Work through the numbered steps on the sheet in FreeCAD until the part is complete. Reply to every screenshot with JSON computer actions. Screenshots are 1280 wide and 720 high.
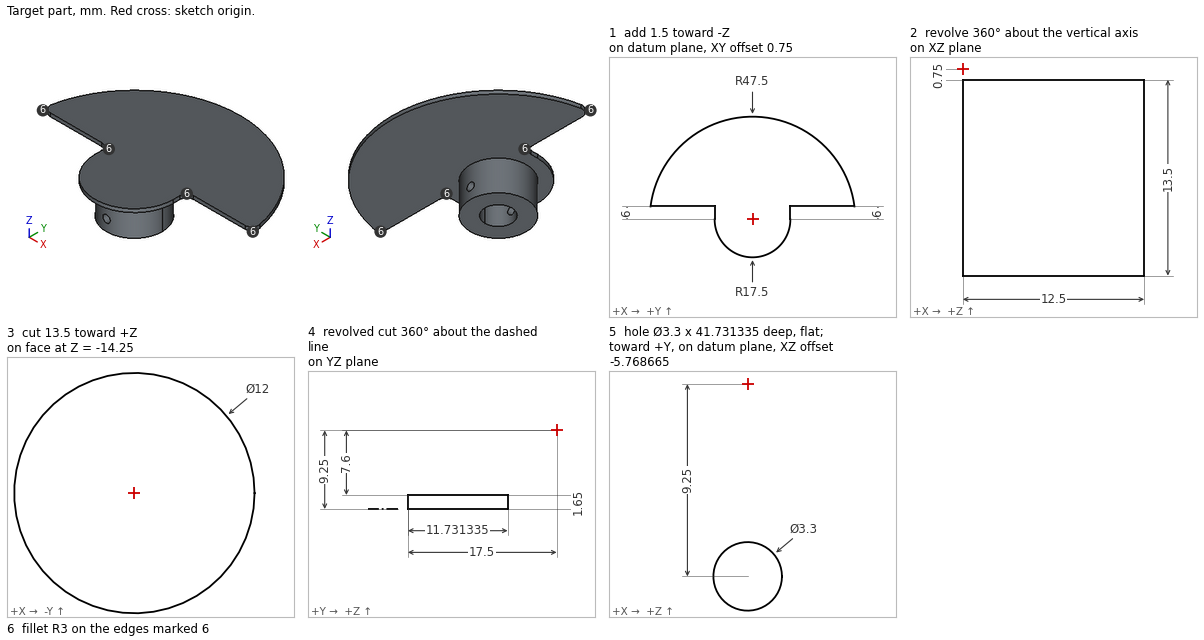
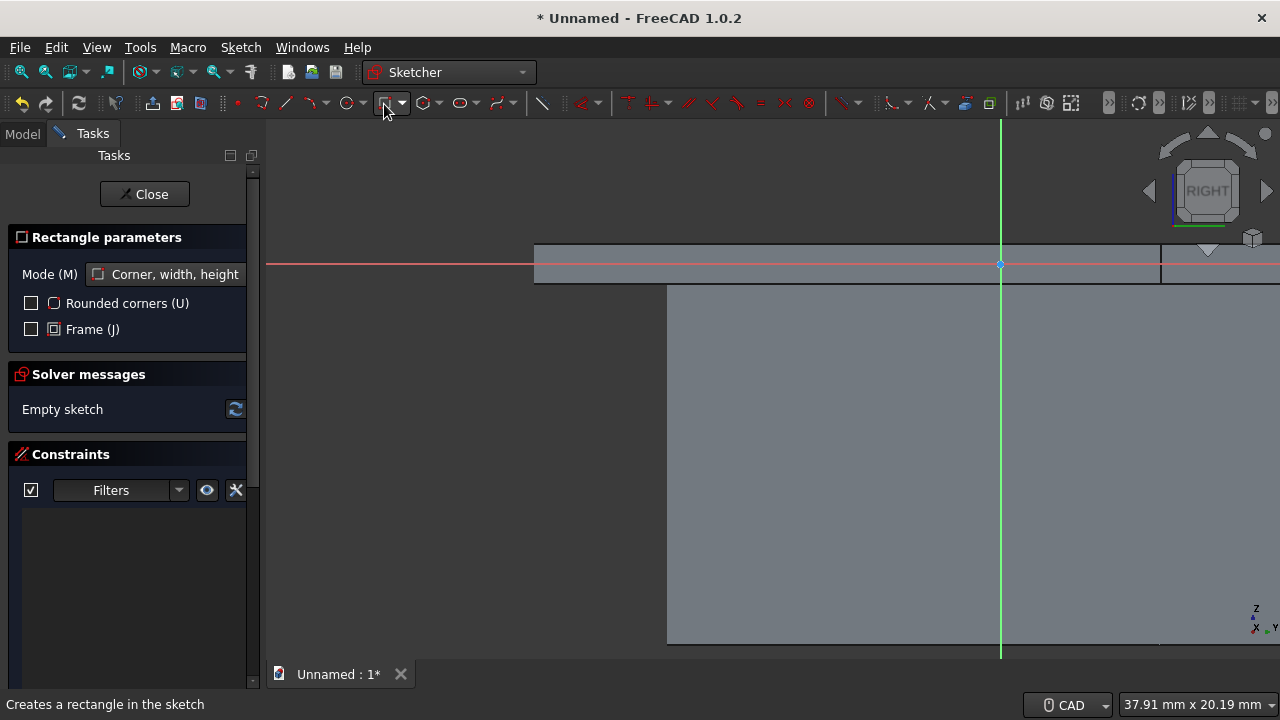
{"action": "left_click", "coordinate": [532, 468]}
{"action": "mouse_move", "coordinate": [846, 512]}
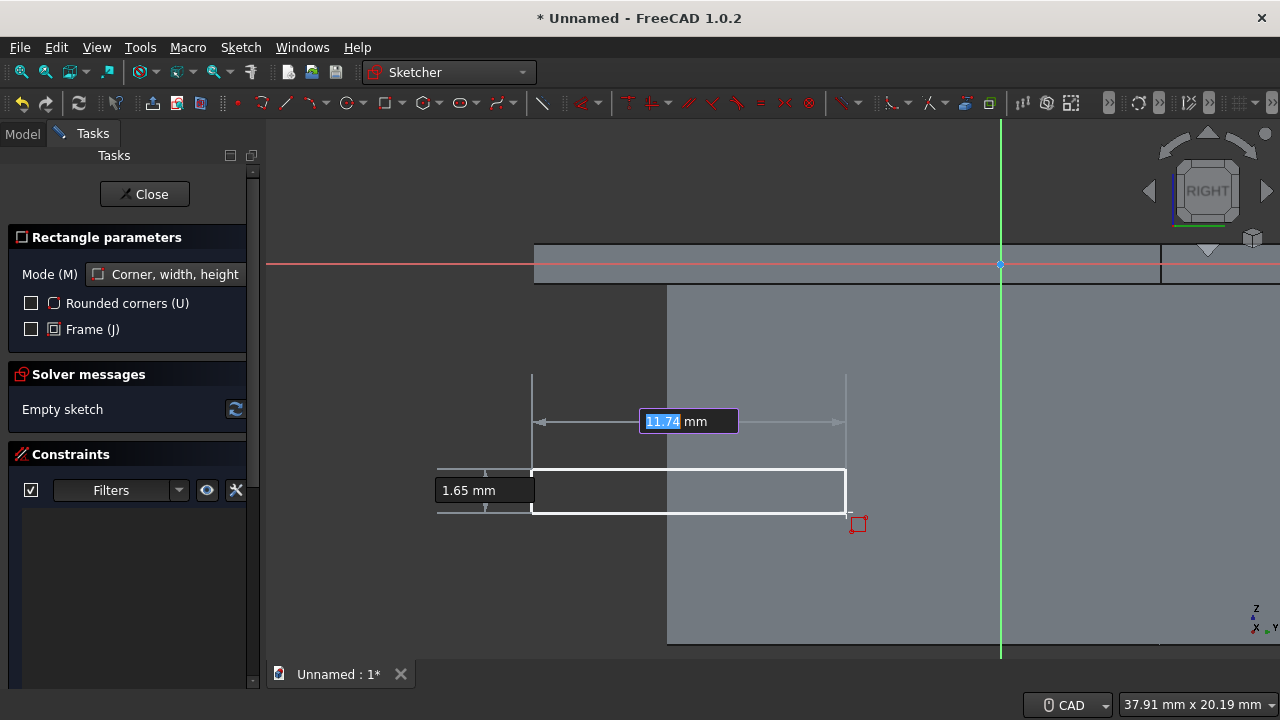
{"action": "type", "text": "11.731335"}
{"action": "key", "text": "Tab"}
{"action": "type", "text": "1.65"}
{"action": "key", "text": "Return"}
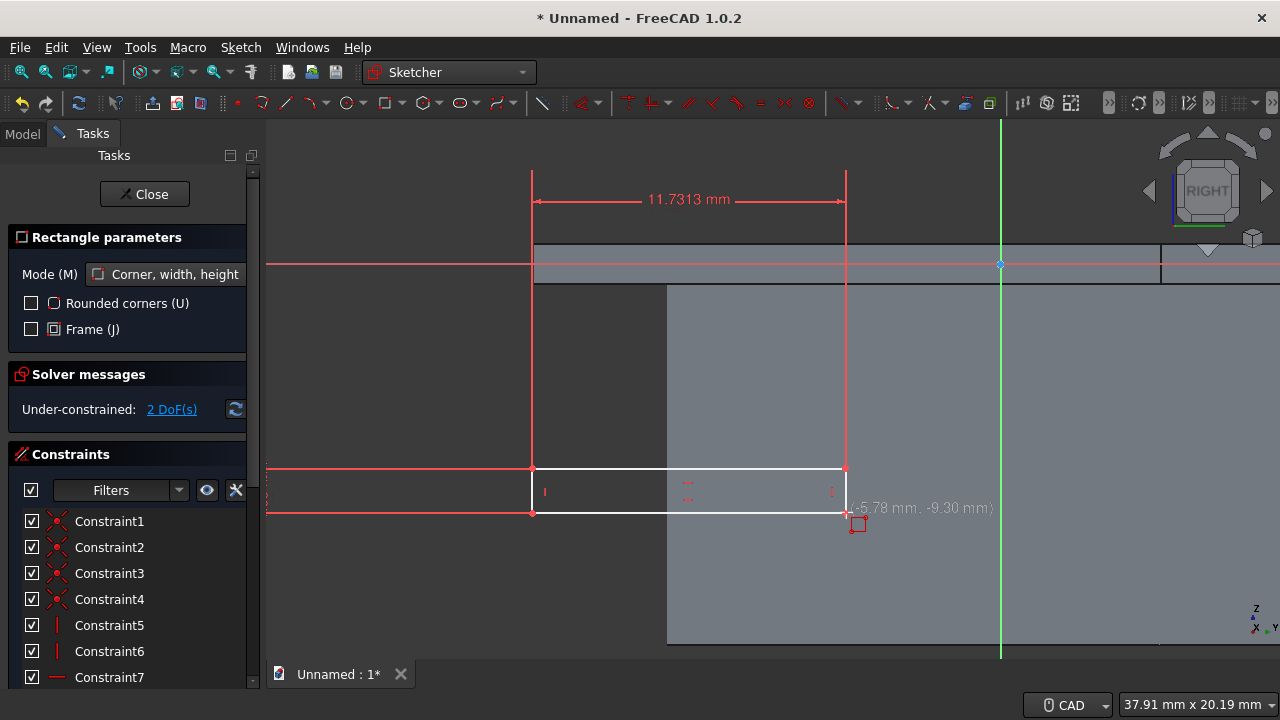
{"action": "left_click", "coordinate": [286, 104]}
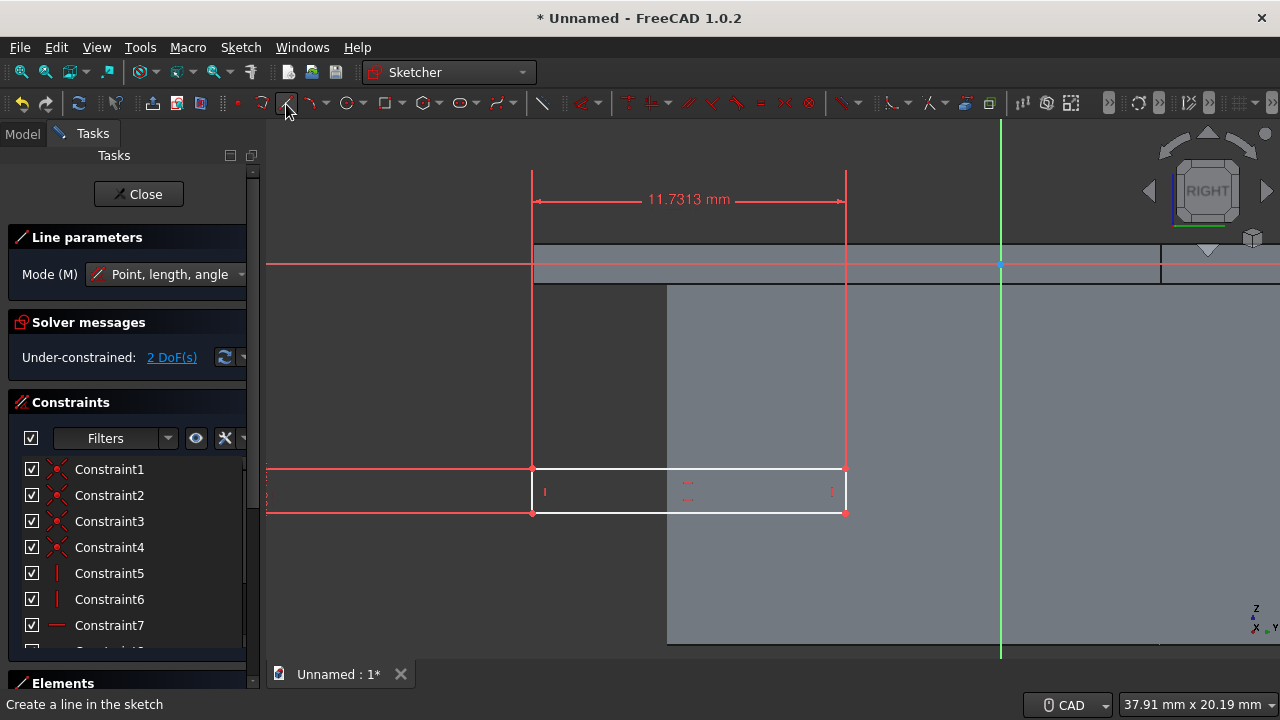
{"action": "left_click", "coordinate": [501, 512]}
{"action": "left_click", "coordinate": [407, 512]}
{"action": "key", "text": "Escape"}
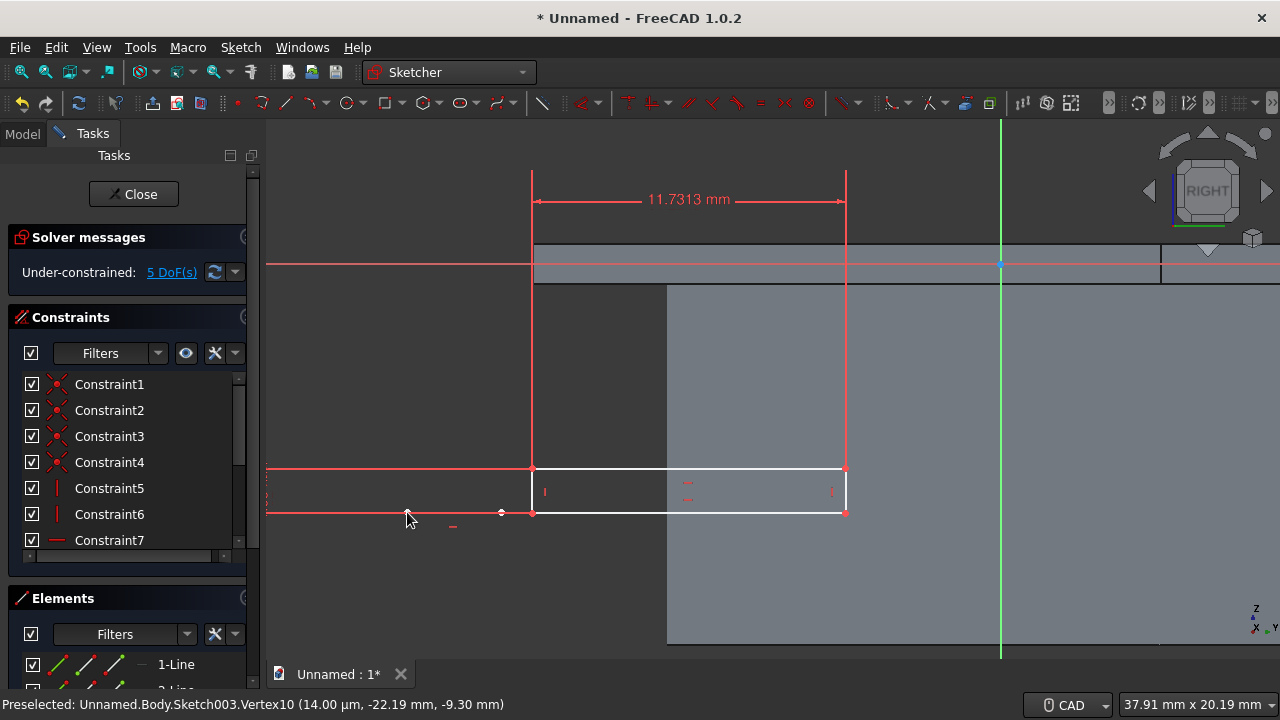
{"action": "left_click", "coordinate": [473, 513]}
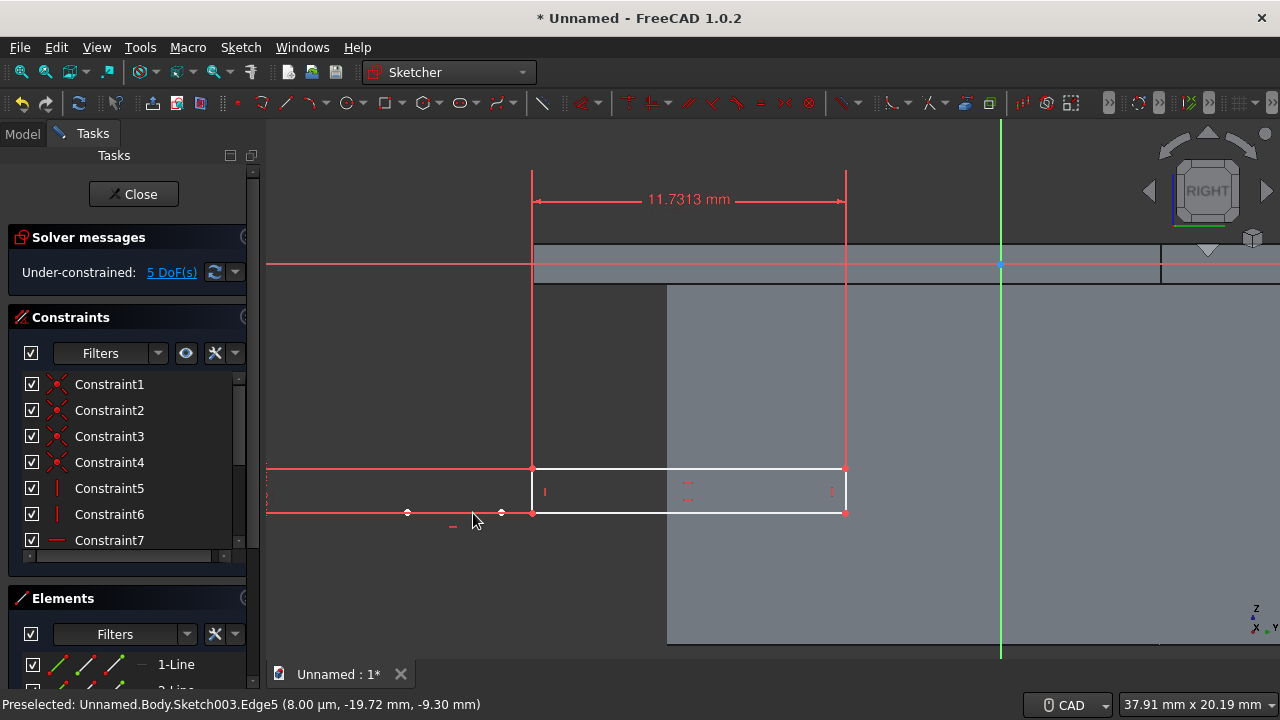
{"action": "key", "text": "g n"}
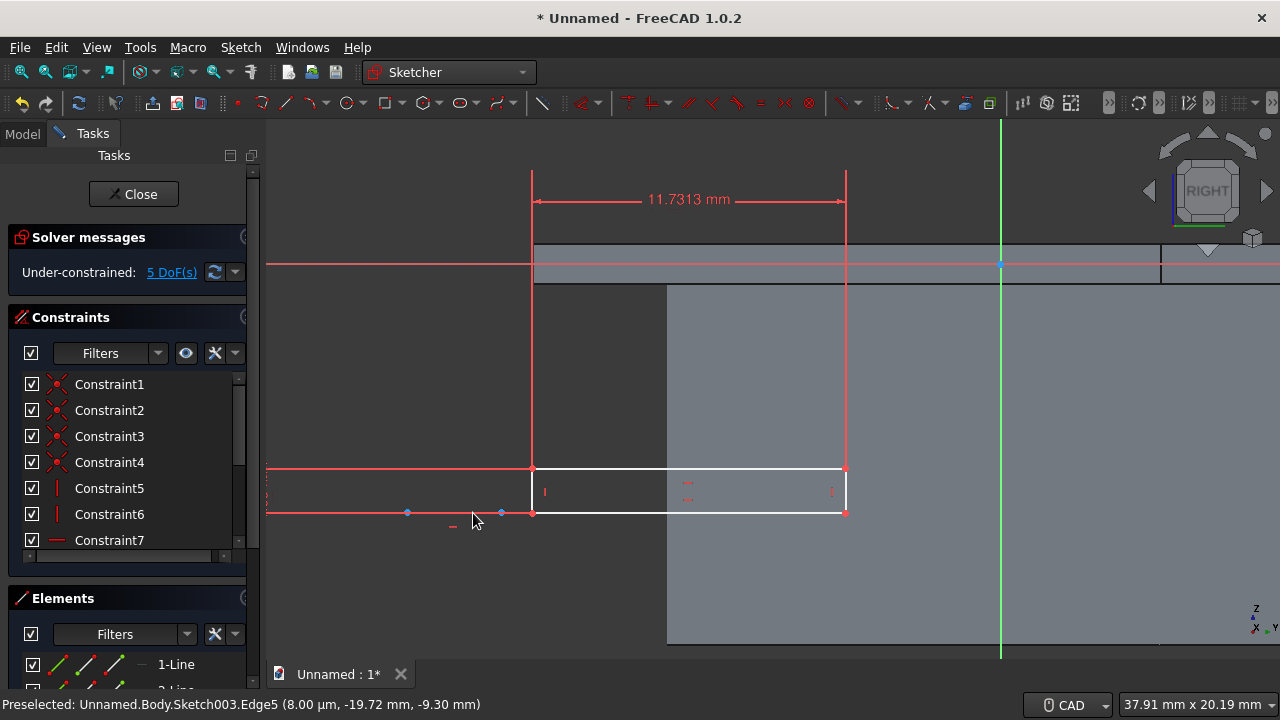
{"action": "left_click", "coordinate": [582, 104]}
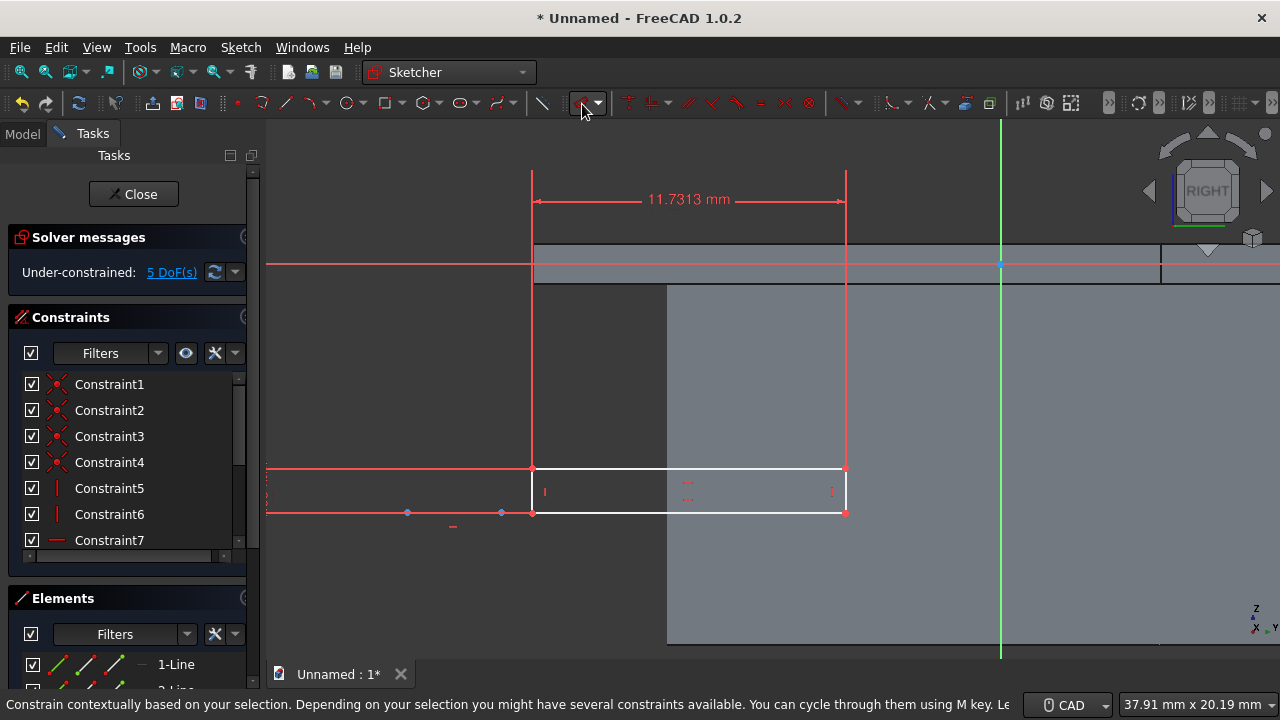
{"action": "left_click", "coordinate": [532, 469]}
{"action": "left_click", "coordinate": [1035, 367]}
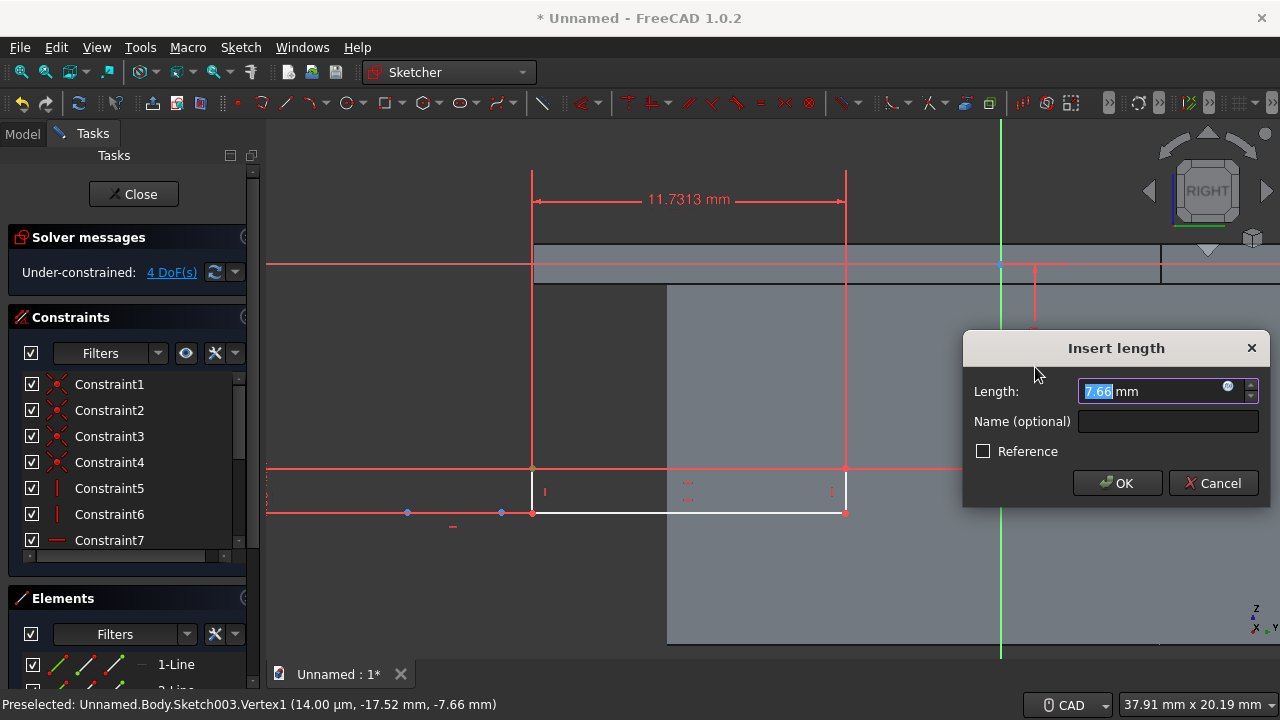
{"action": "type", "text": "7.6"}
{"action": "key", "text": "Return"}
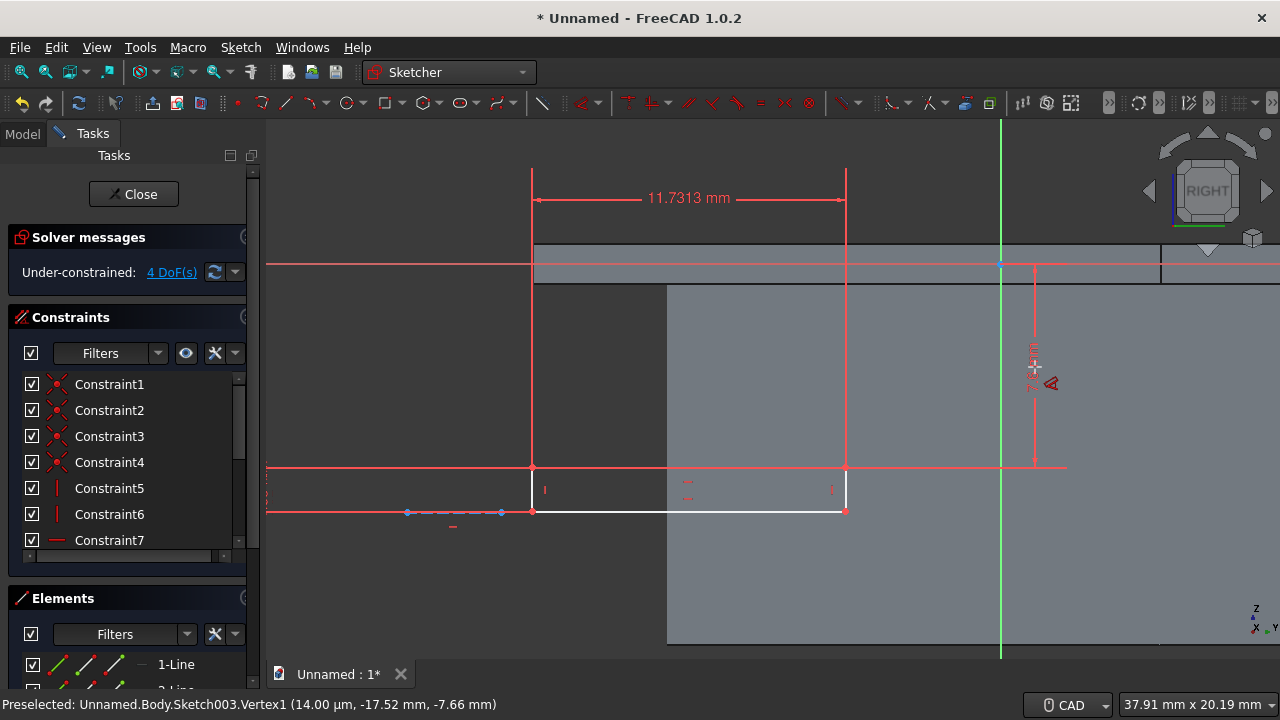
{"action": "left_click", "coordinate": [532, 468]}
{"action": "left_click", "coordinate": [766, 230]}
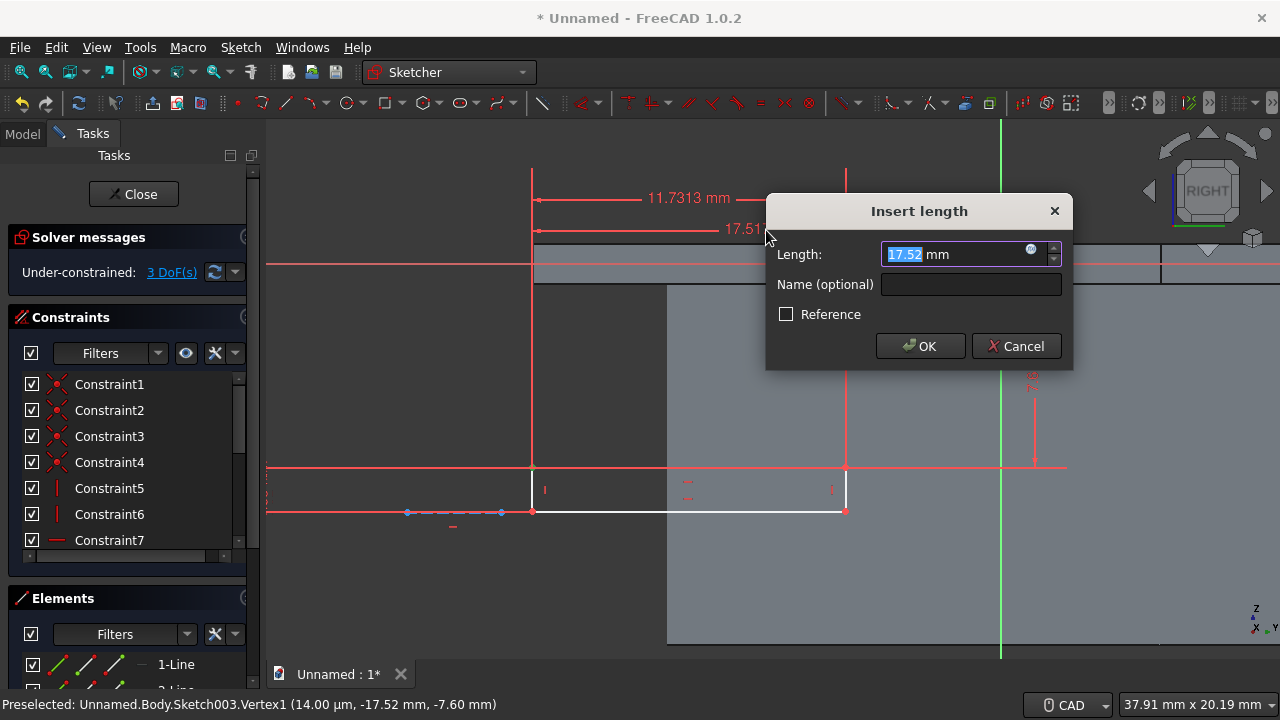
{"action": "type", "text": "17.5"}
{"action": "key", "text": "Return"}